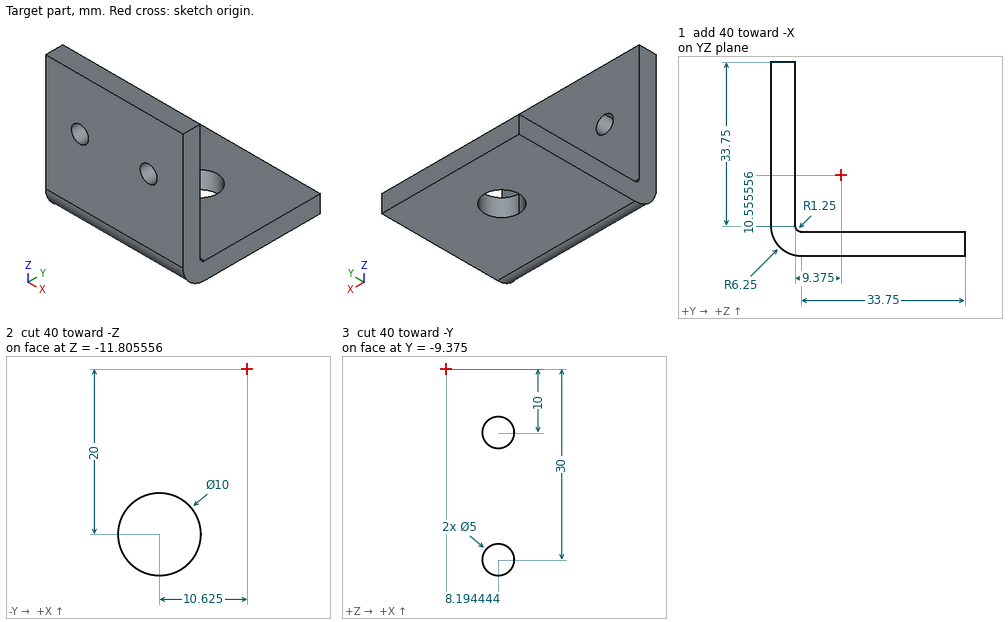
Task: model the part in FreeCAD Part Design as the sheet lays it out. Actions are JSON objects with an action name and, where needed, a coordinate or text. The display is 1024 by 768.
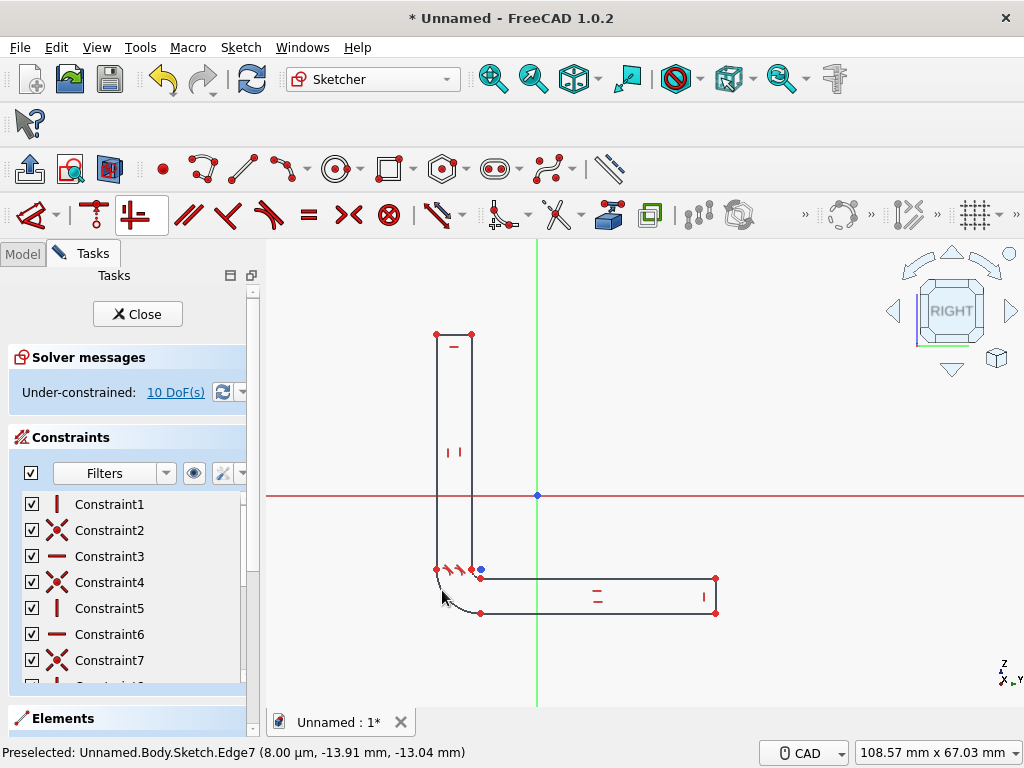
{"action": "left_click", "coordinate": [551, 614]}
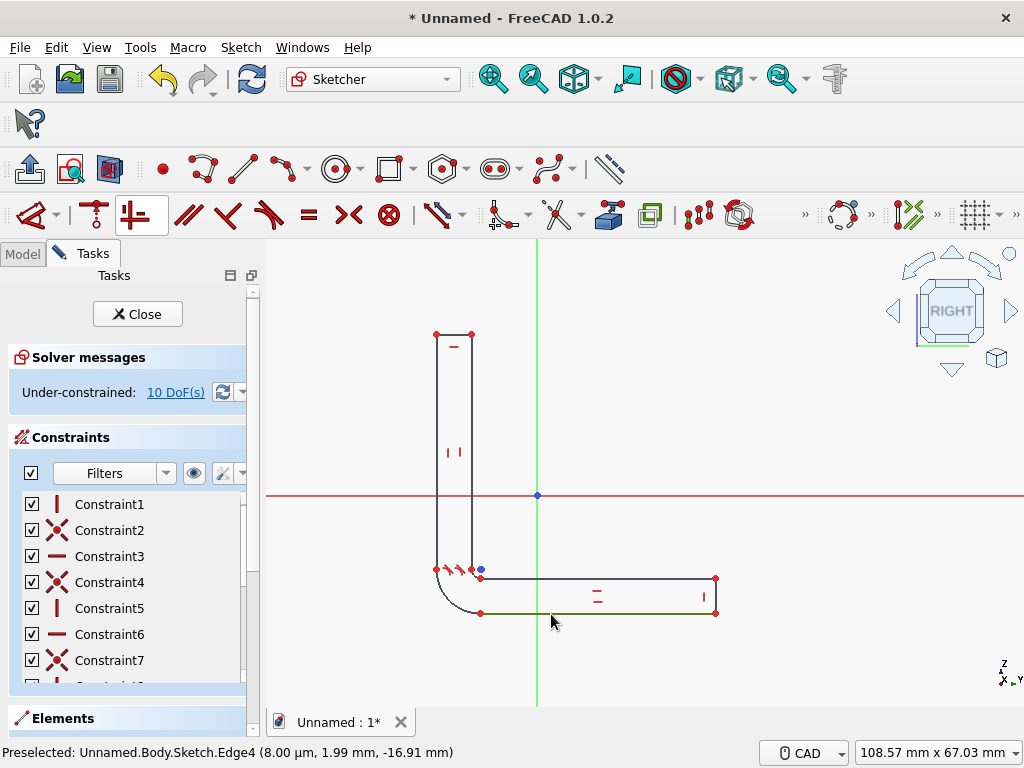
{"action": "left_click", "coordinate": [442, 590]}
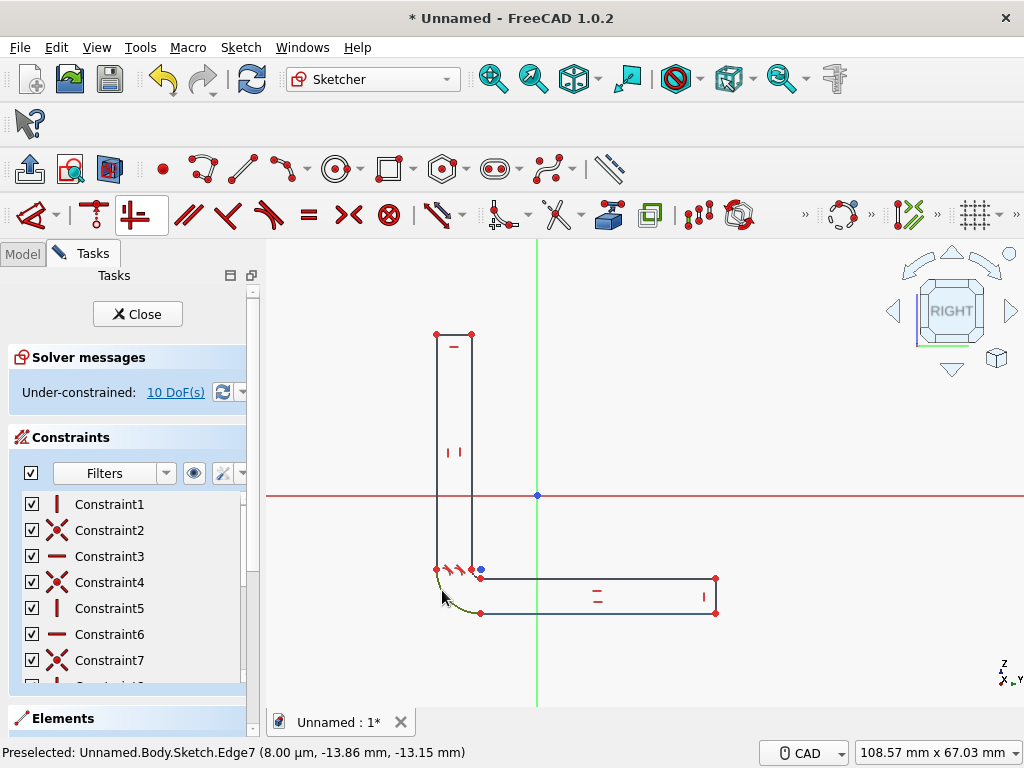
{"action": "left_click", "coordinate": [270, 216]}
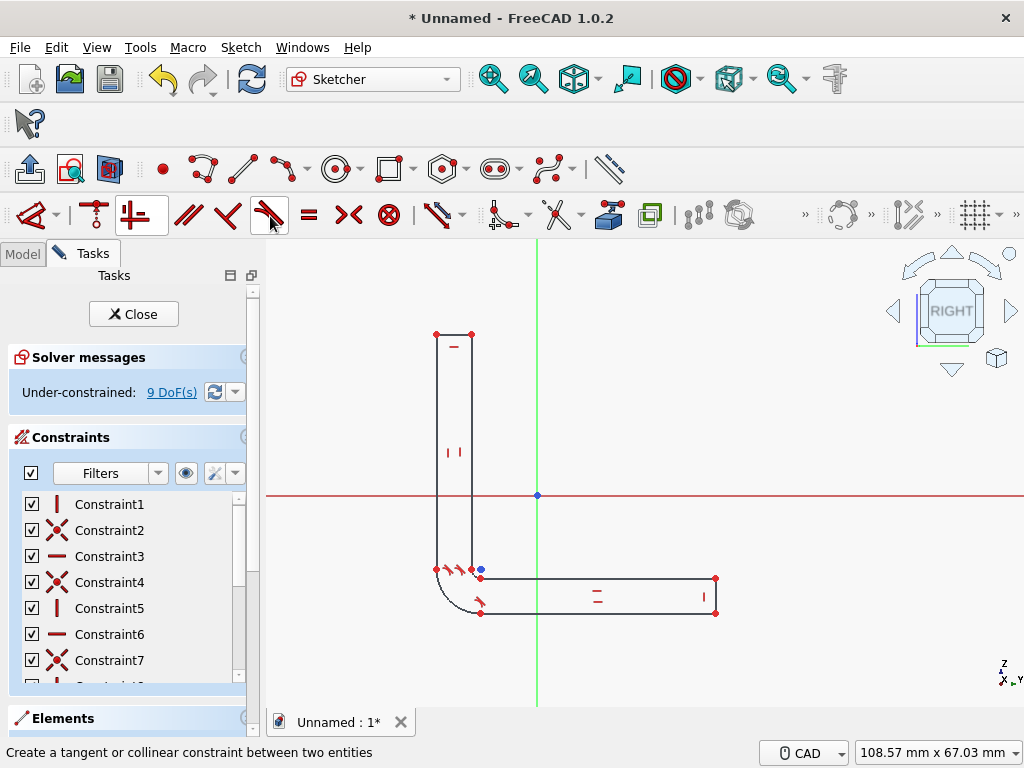
{"action": "left_click", "coordinate": [645, 579]}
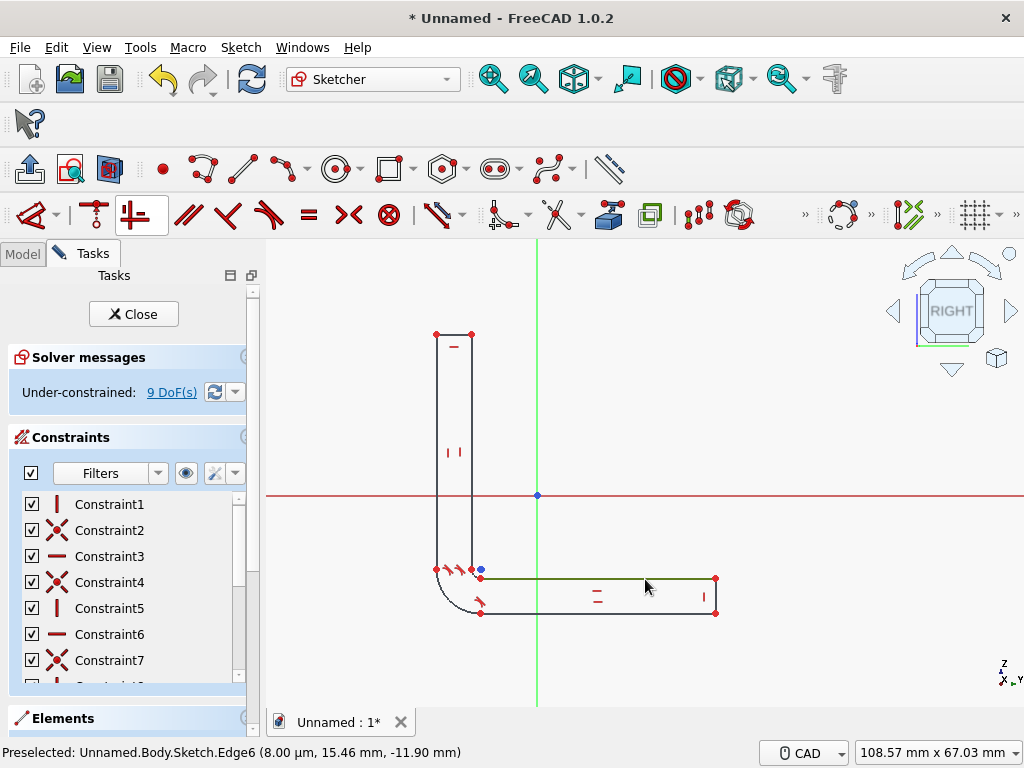
{"action": "scroll", "coordinate": [474, 575], "scroll_direction": "up", "scroll_amount": 4}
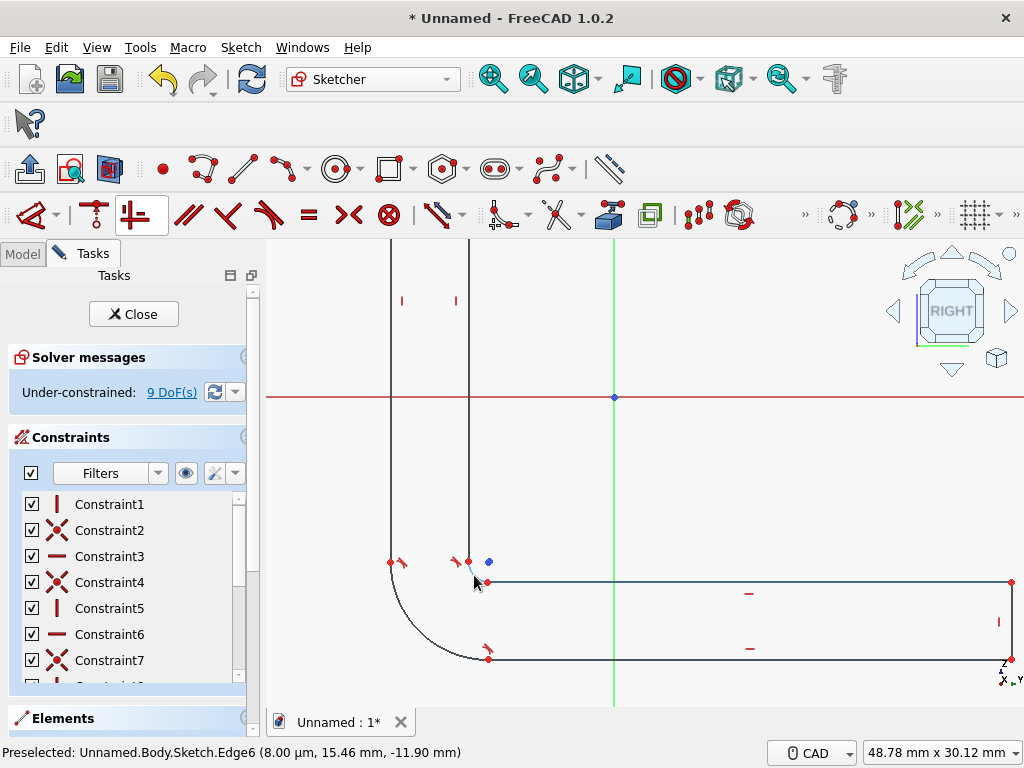
{"action": "left_click", "coordinate": [474, 575]}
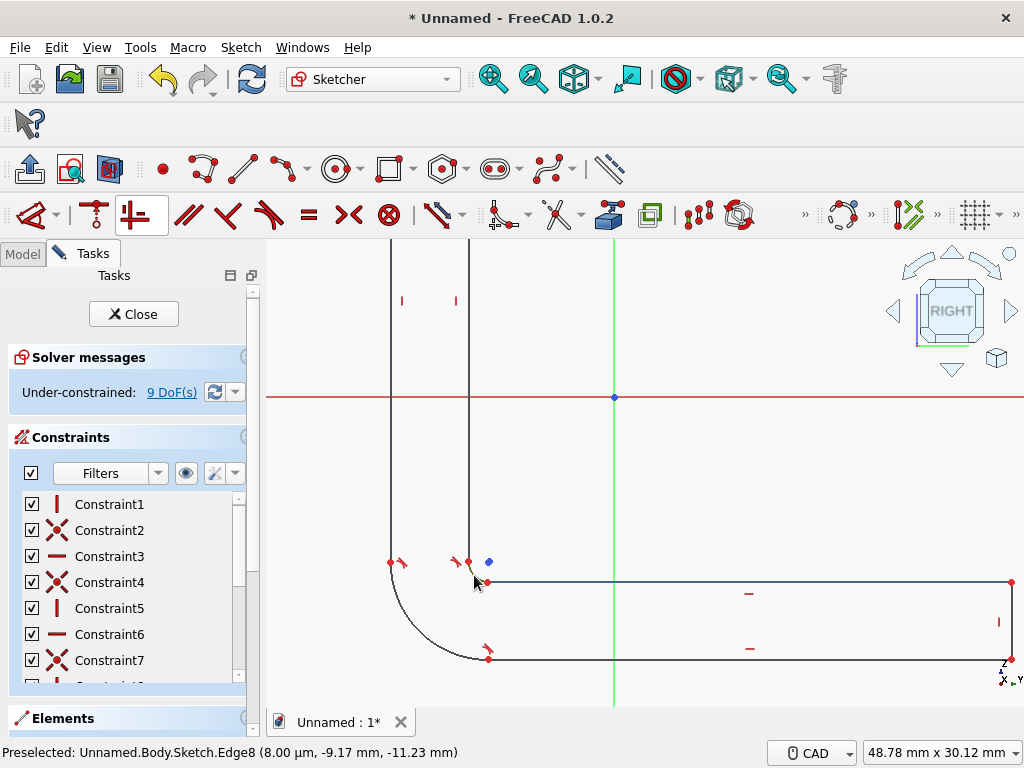
{"action": "key", "text": "t"}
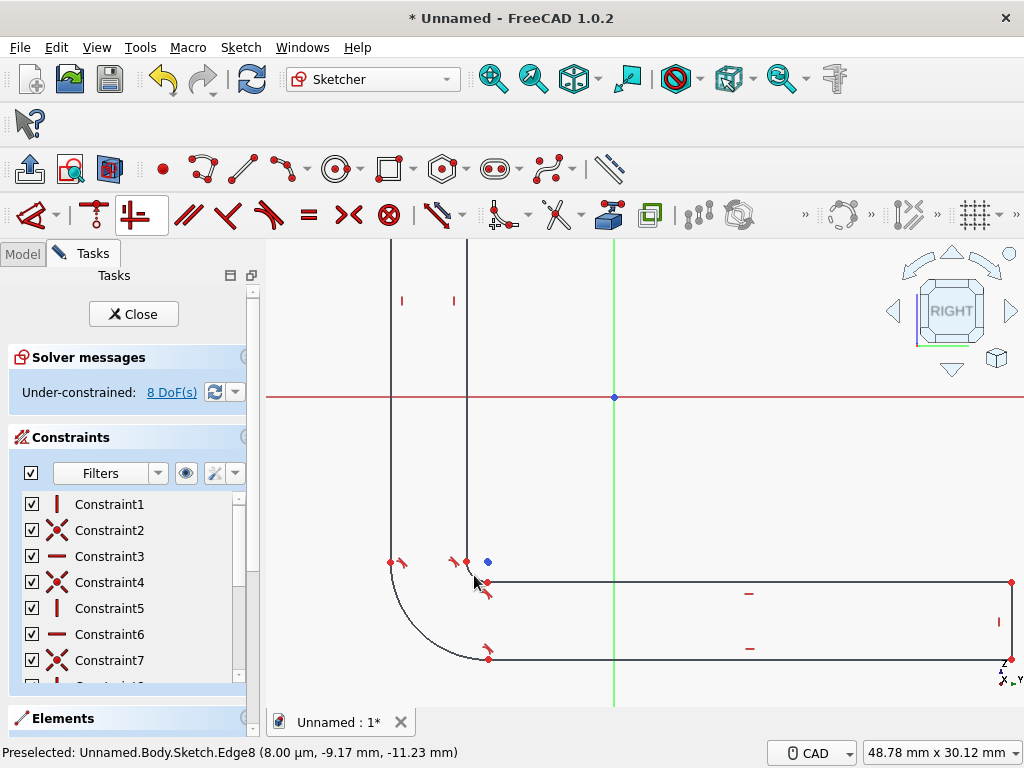
{"action": "left_click", "coordinate": [401, 607]}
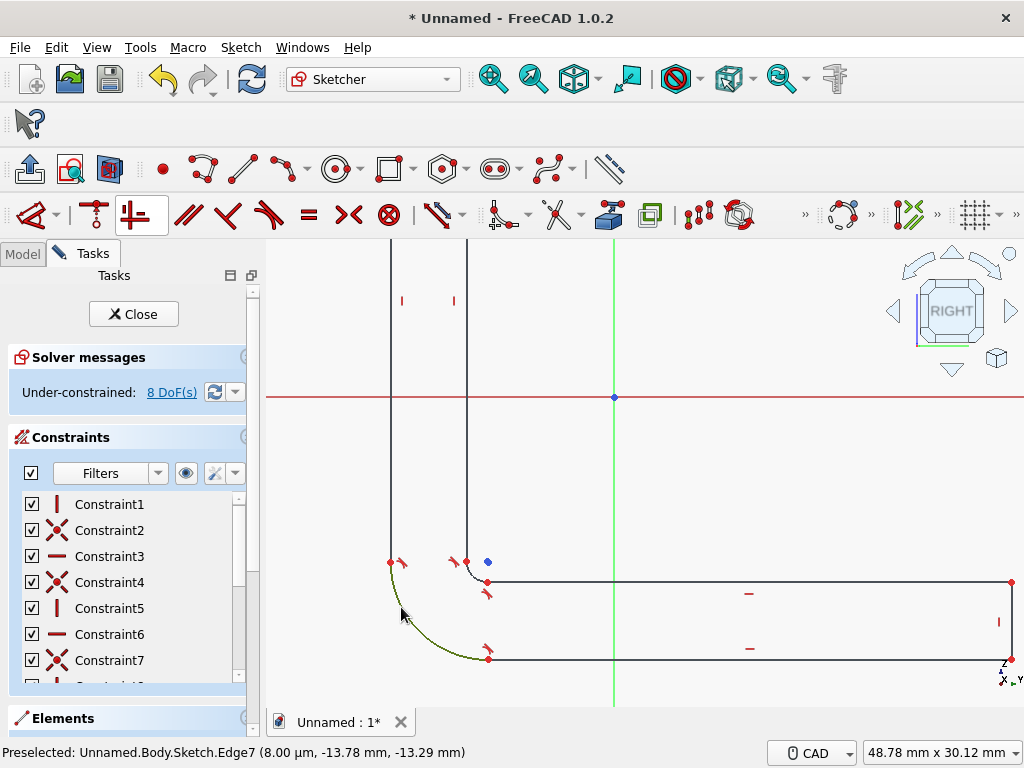
{"action": "scroll", "coordinate": [469, 571], "scroll_direction": "up", "scroll_amount": 2}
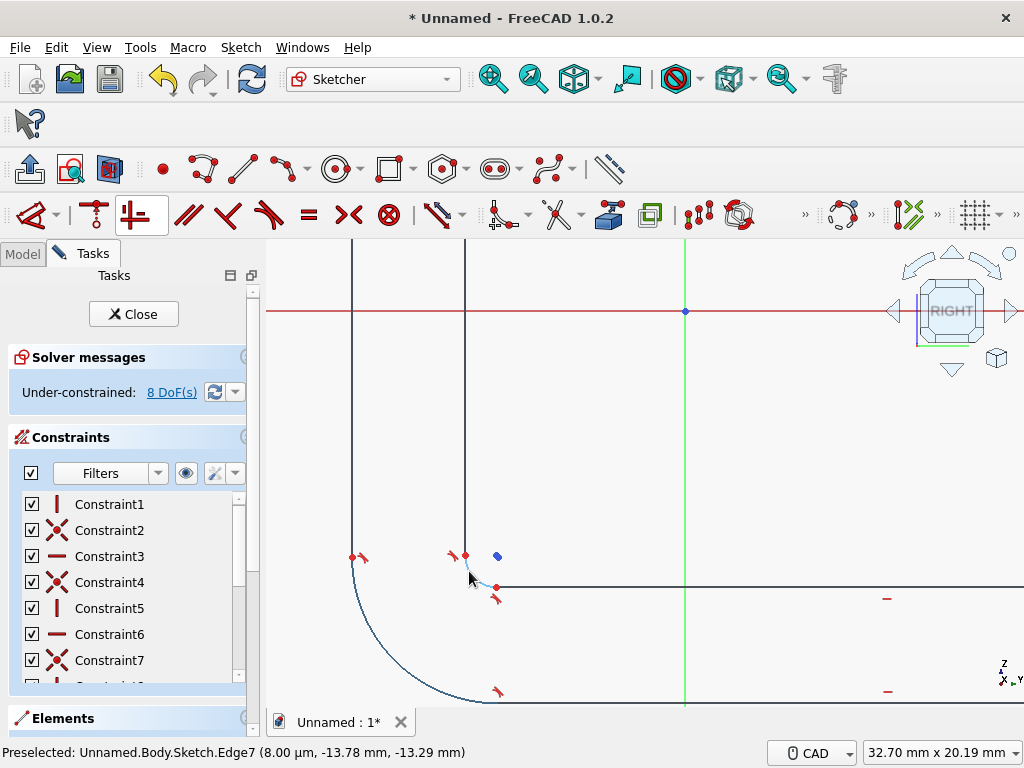
{"action": "left_click", "coordinate": [469, 570]}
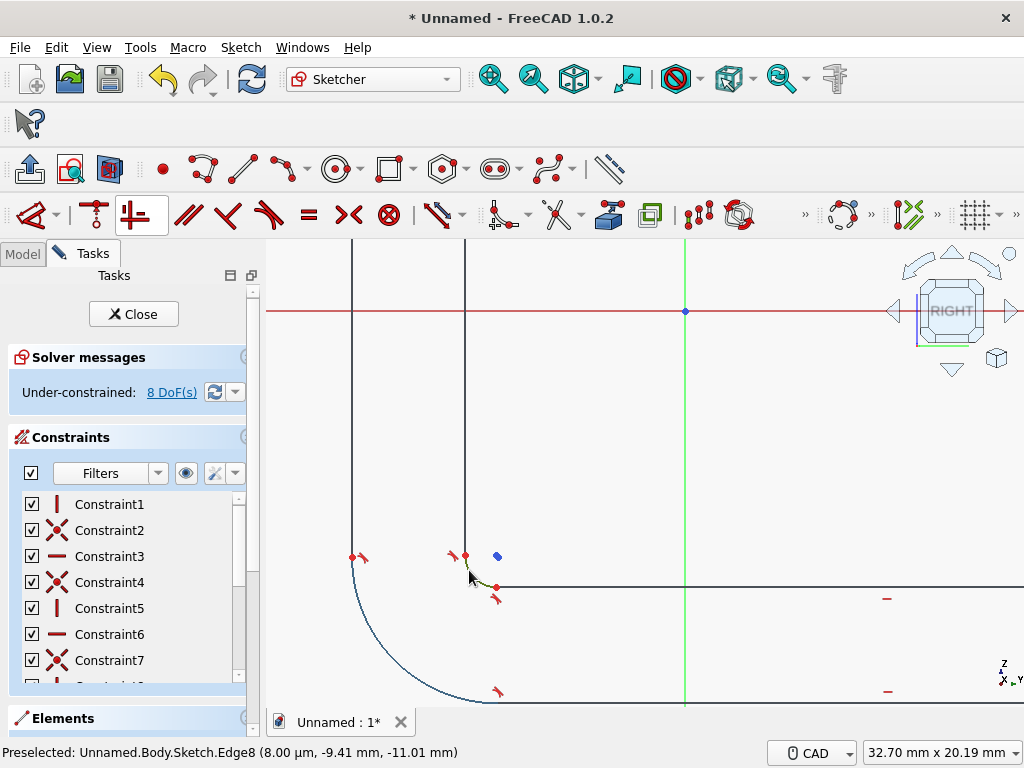
{"action": "key", "text": "c"}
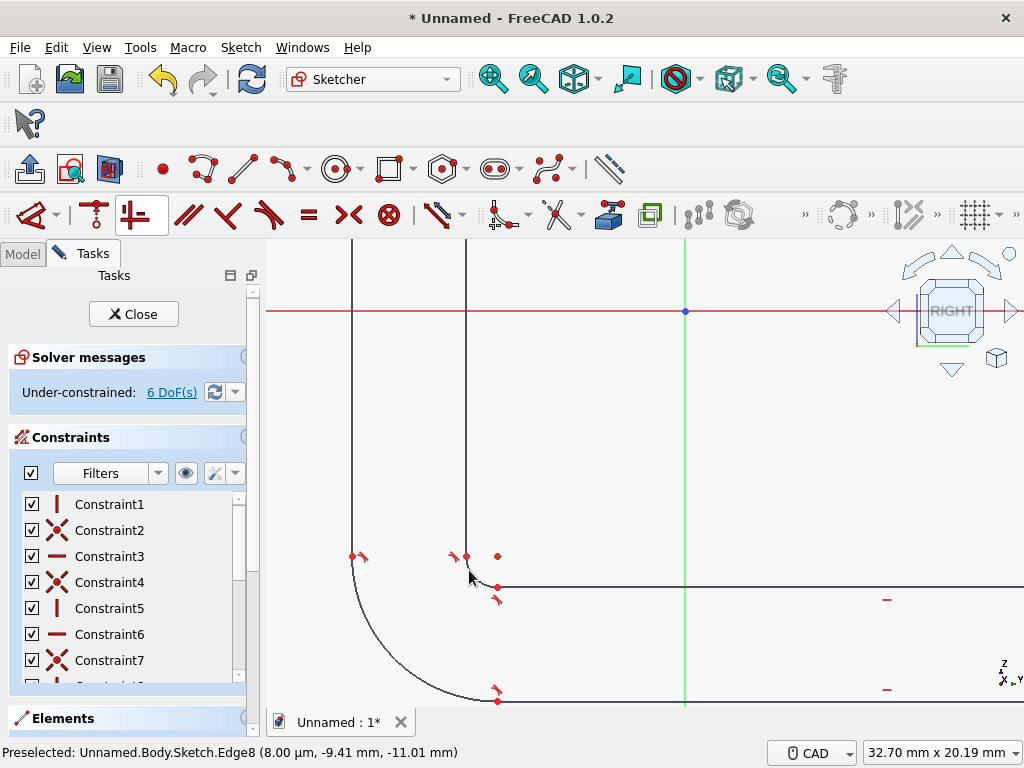
{"action": "left_click", "coordinate": [32, 216]}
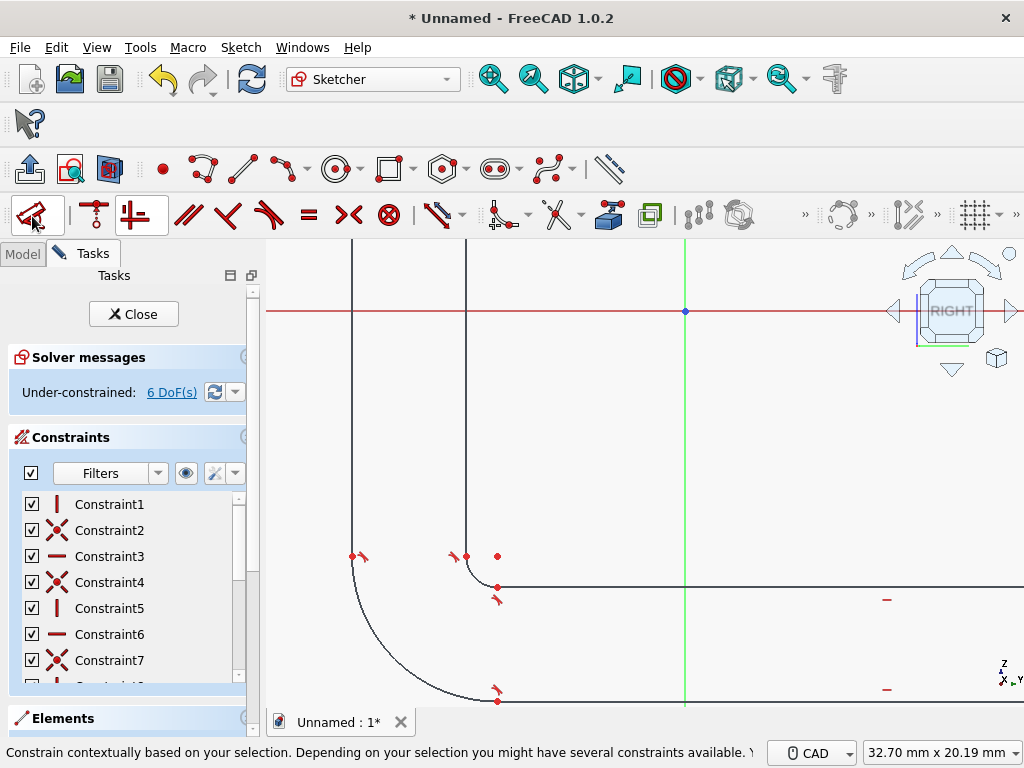
{"action": "left_click", "coordinate": [368, 622]}
{"action": "left_click", "coordinate": [339, 637]}